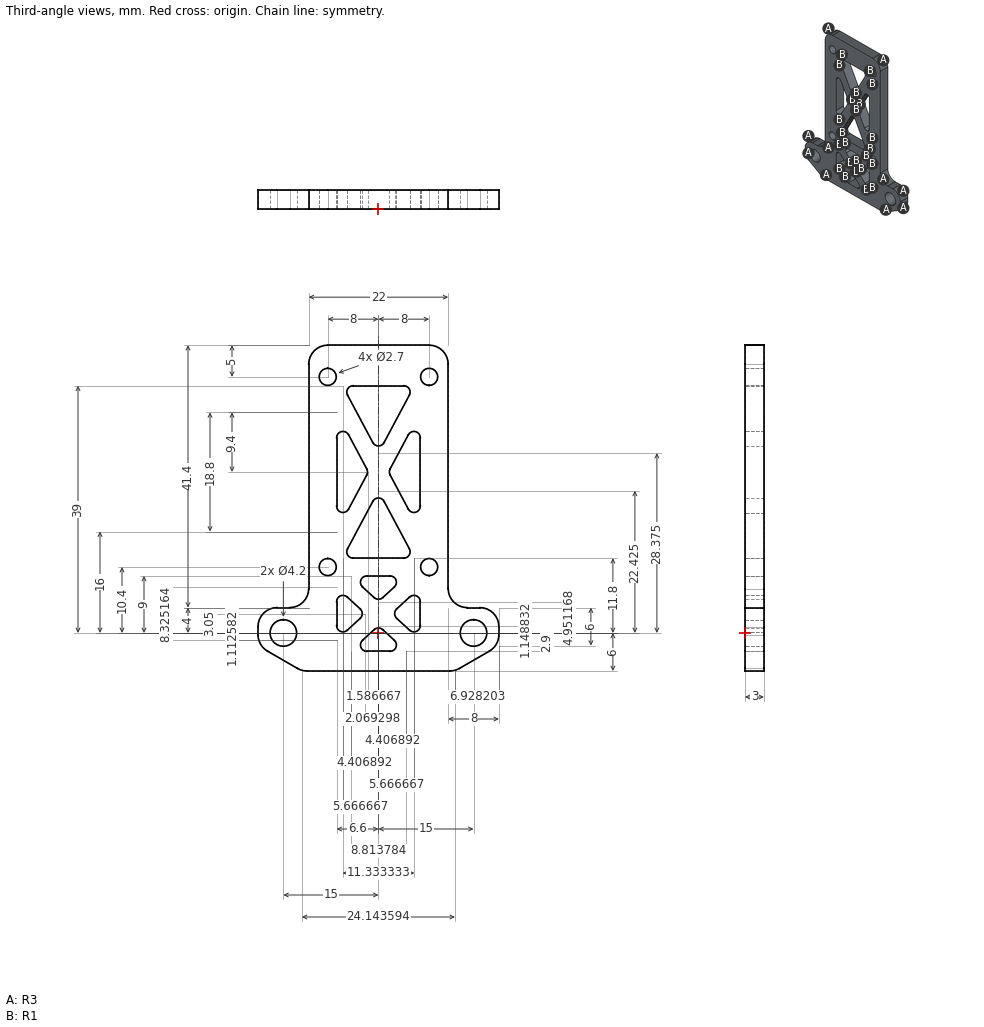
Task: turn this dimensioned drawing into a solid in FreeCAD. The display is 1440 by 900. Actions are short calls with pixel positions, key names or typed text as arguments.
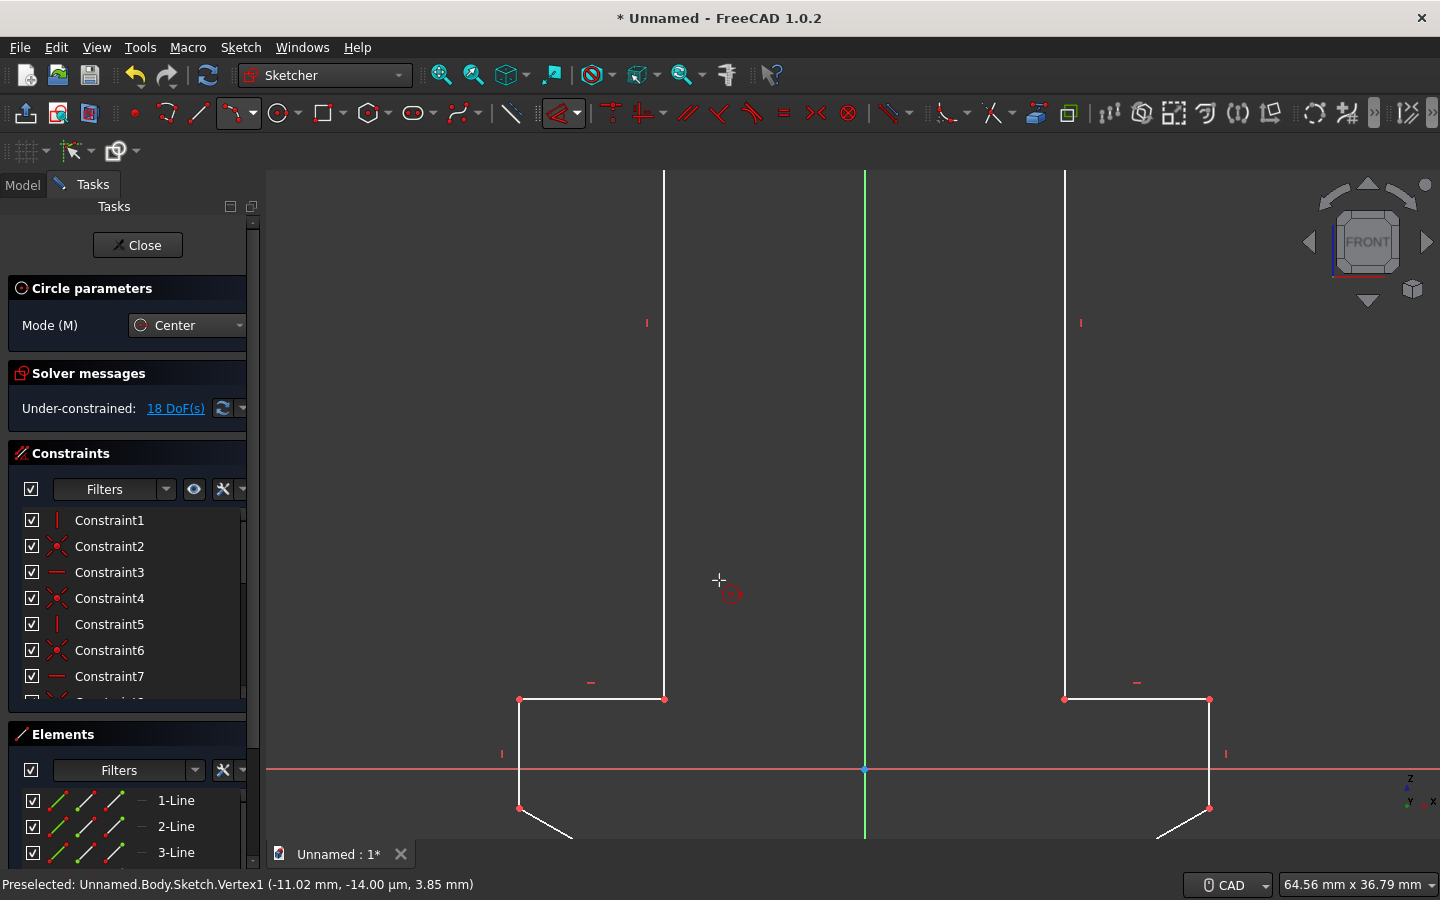
click(719, 580)
click(736, 563)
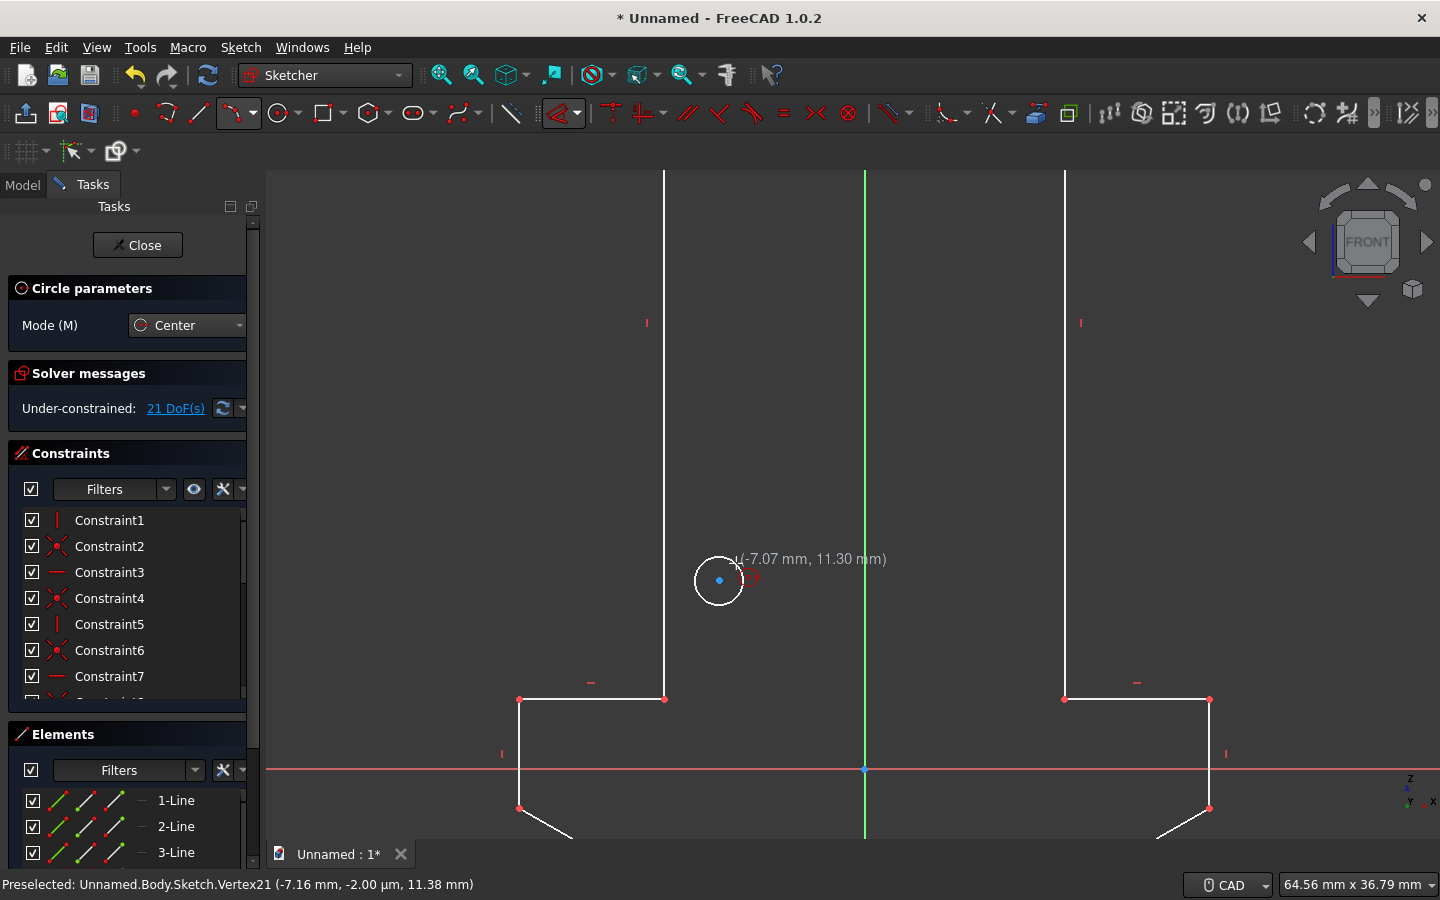
click(592, 769)
click(619, 742)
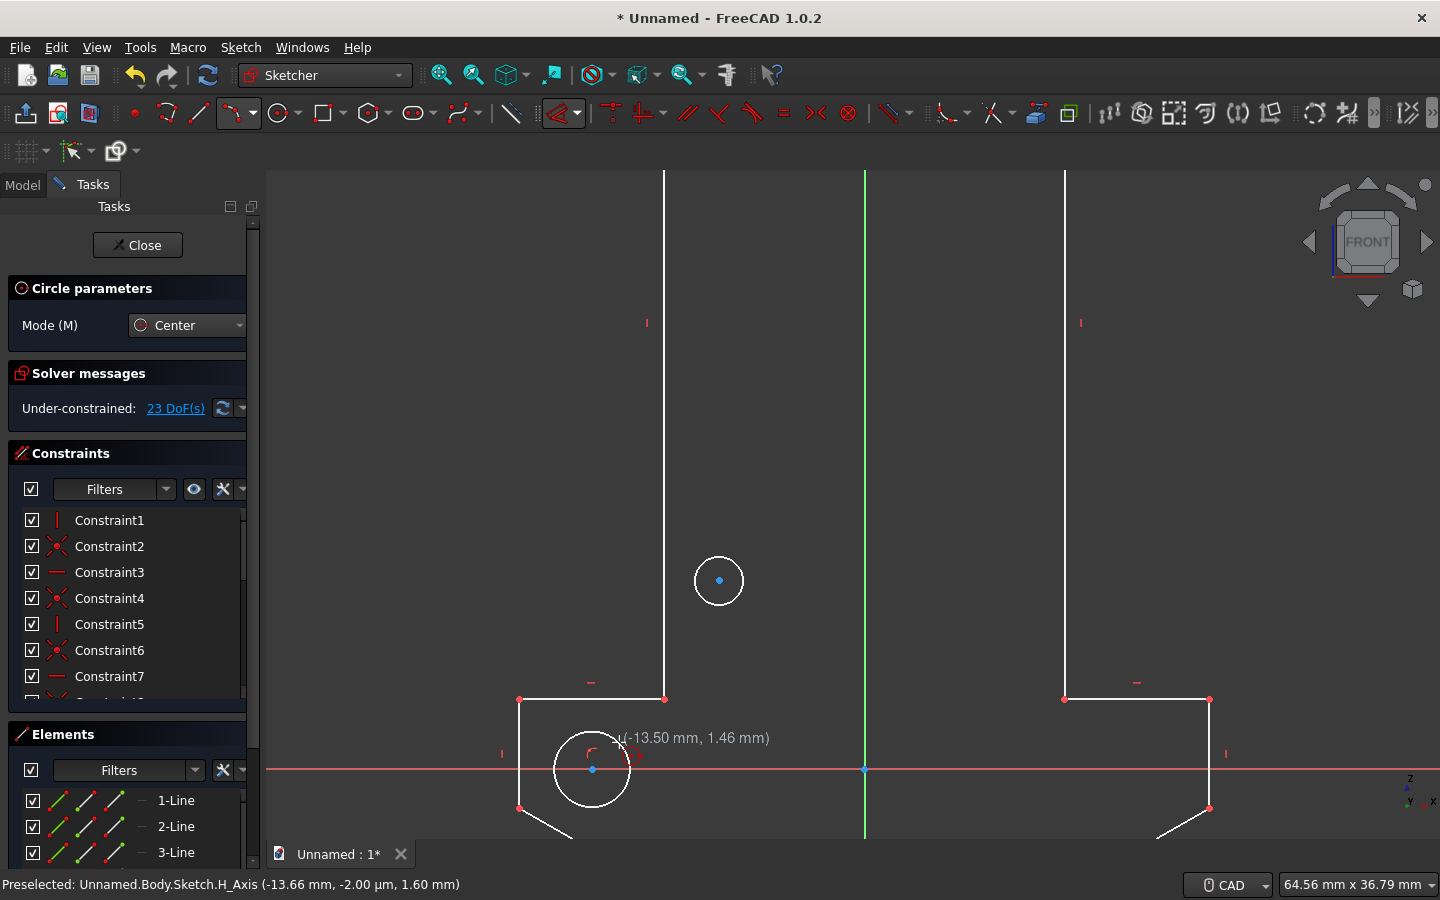
click(1010, 580)
click(1027, 563)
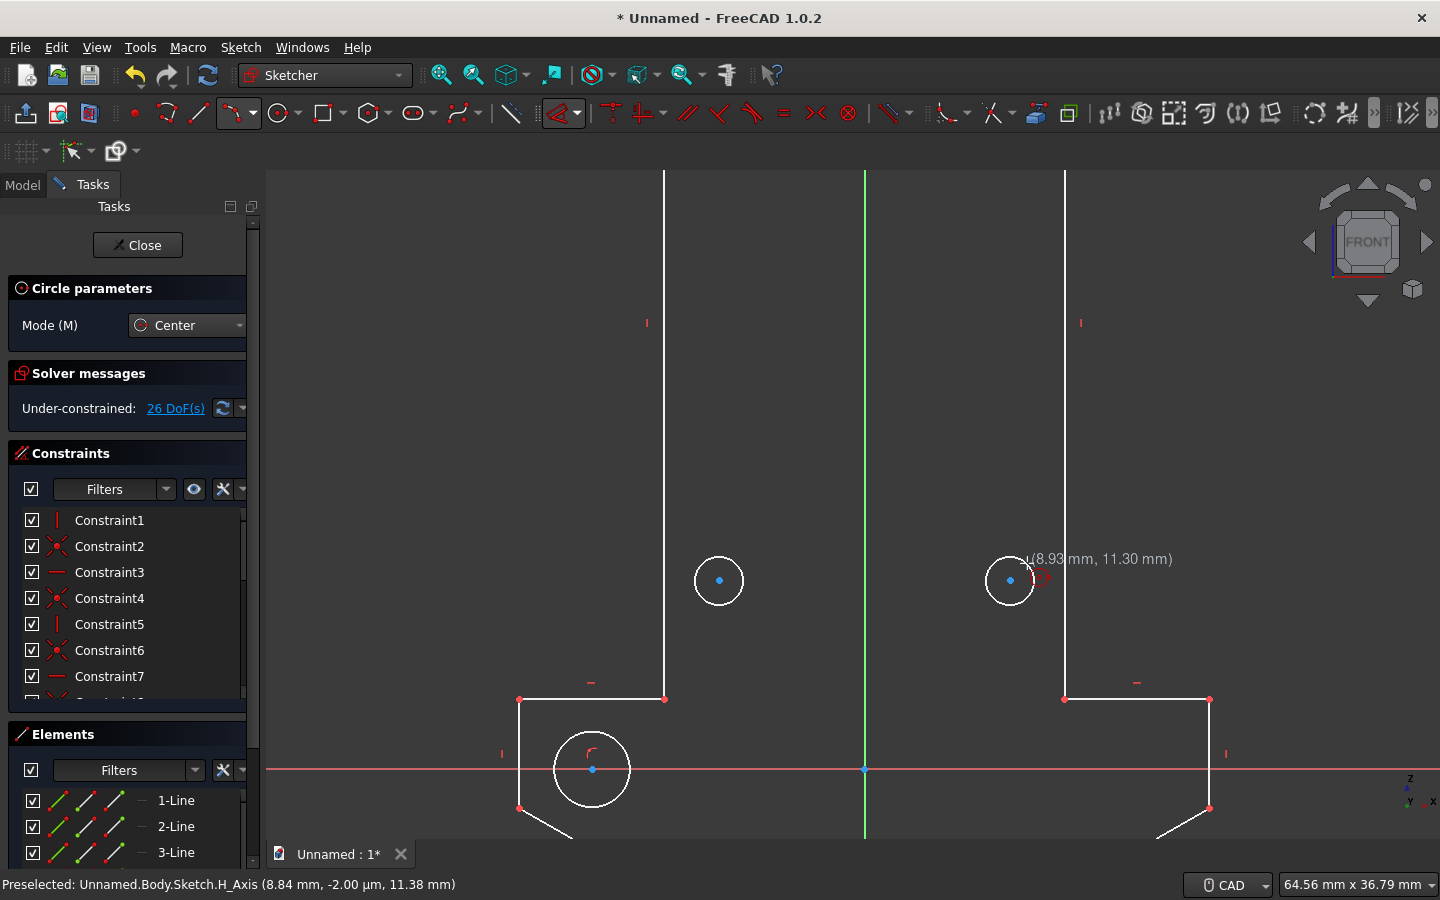
click(1137, 769)
click(1164, 742)
key(Escape)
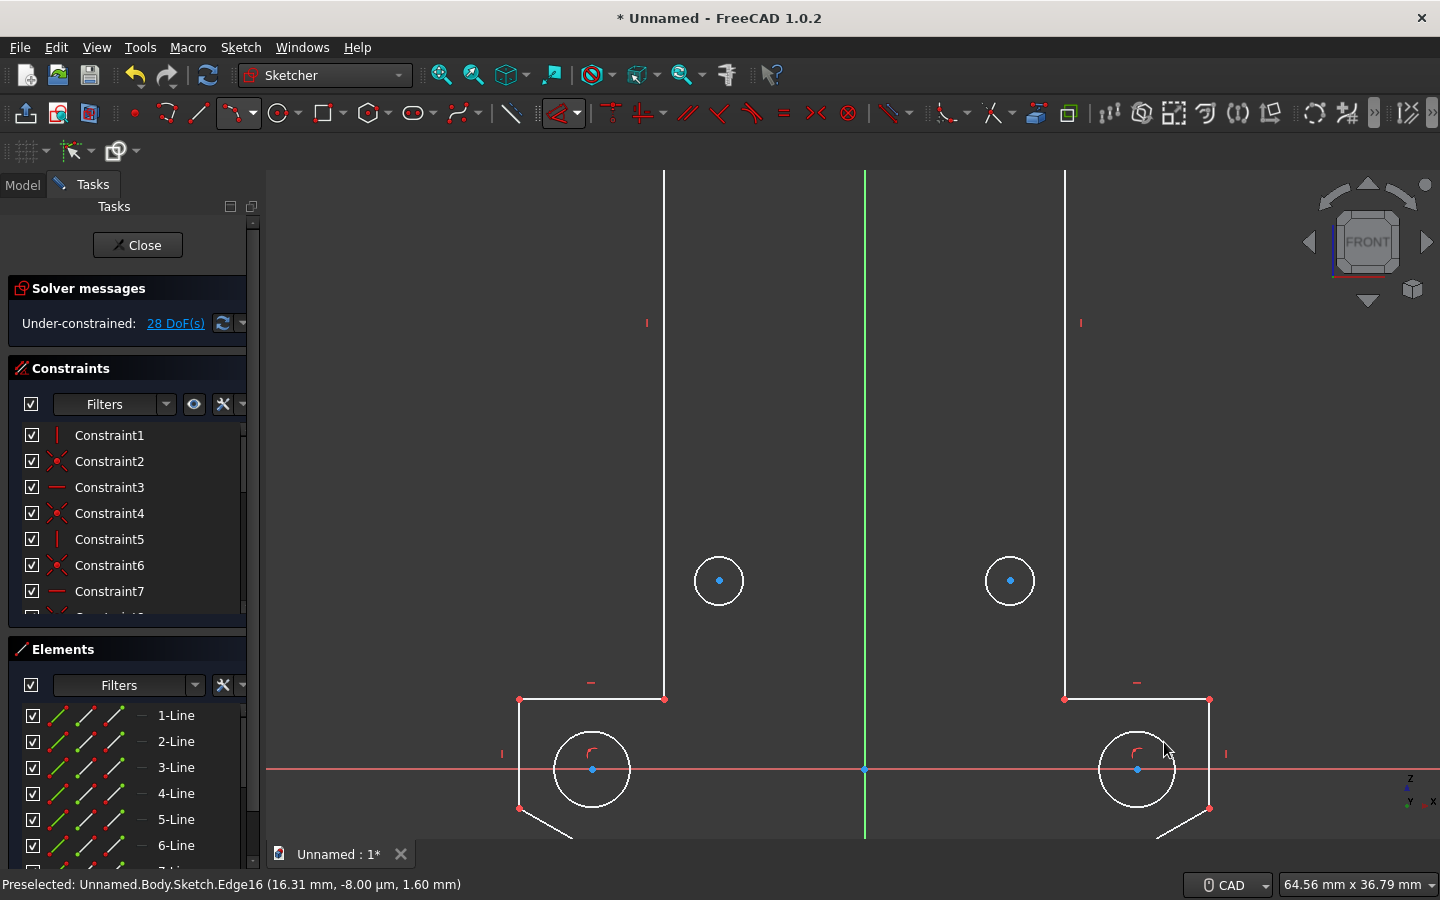
scroll(719, 581, down, 4)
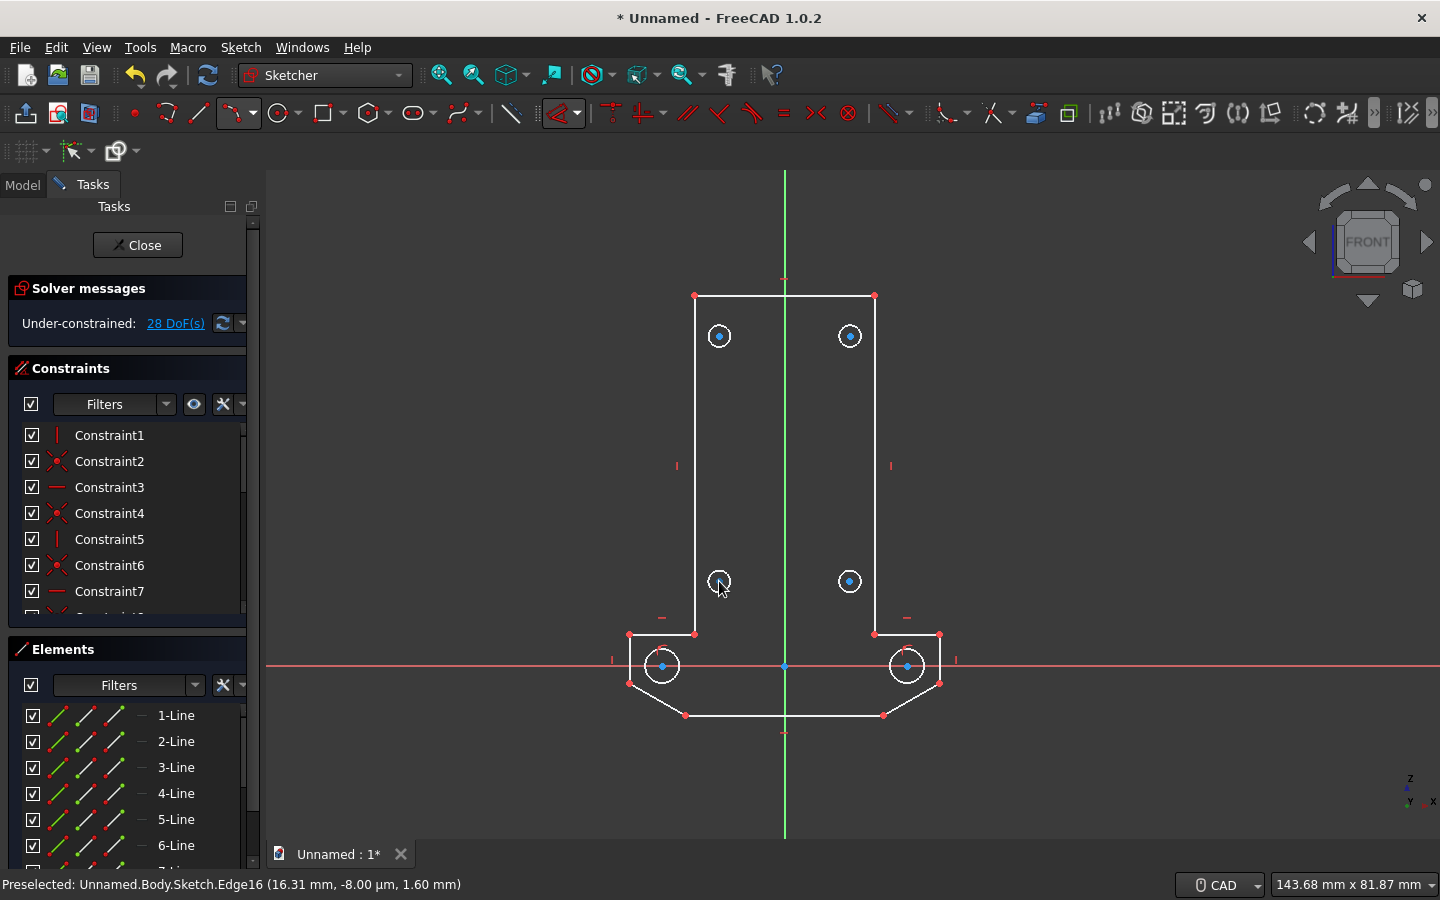
scroll(727, 328, up, 2)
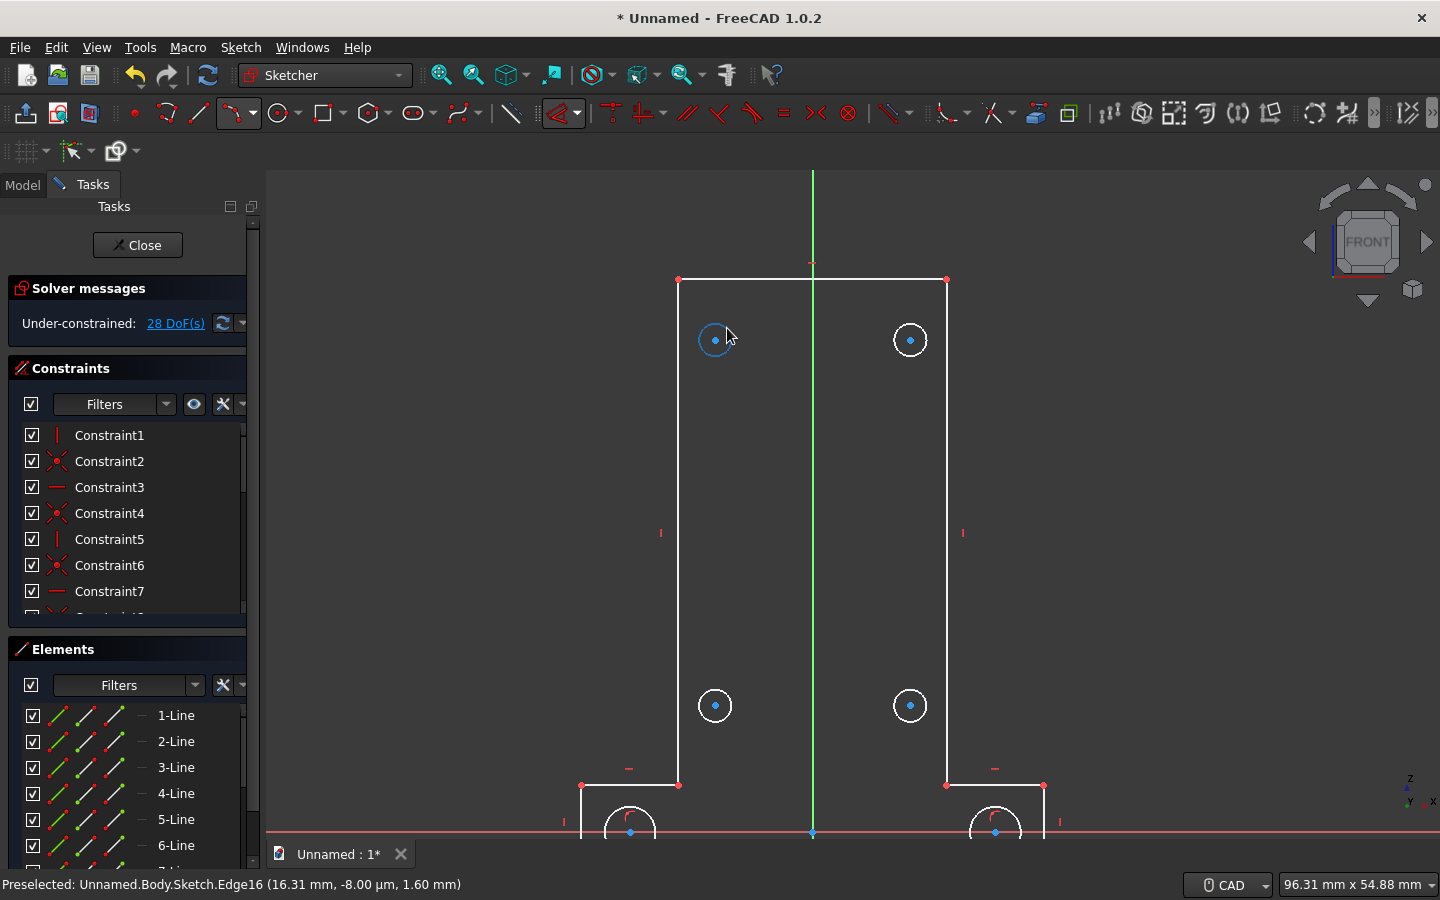
click(727, 329)